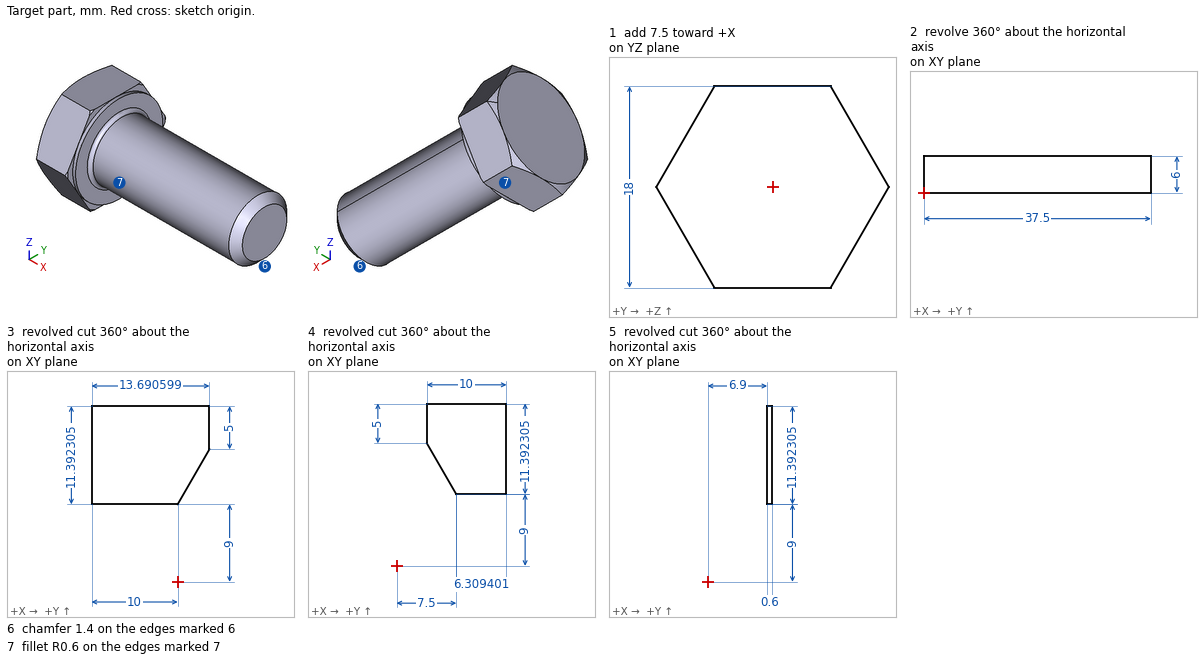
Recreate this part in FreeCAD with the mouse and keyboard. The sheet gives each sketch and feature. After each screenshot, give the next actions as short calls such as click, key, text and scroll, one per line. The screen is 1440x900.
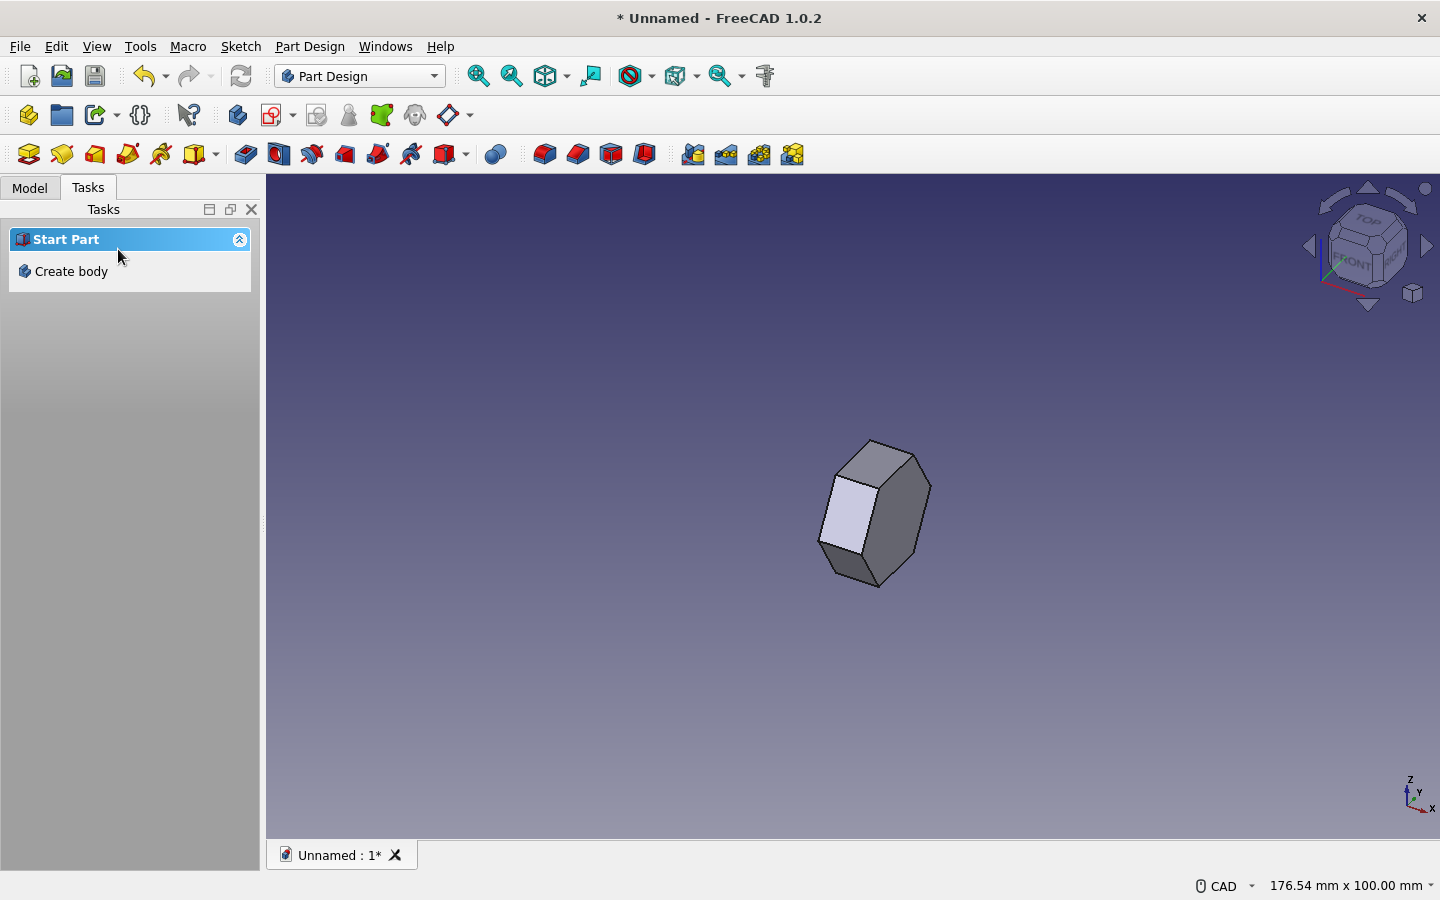
key(v)
key(f)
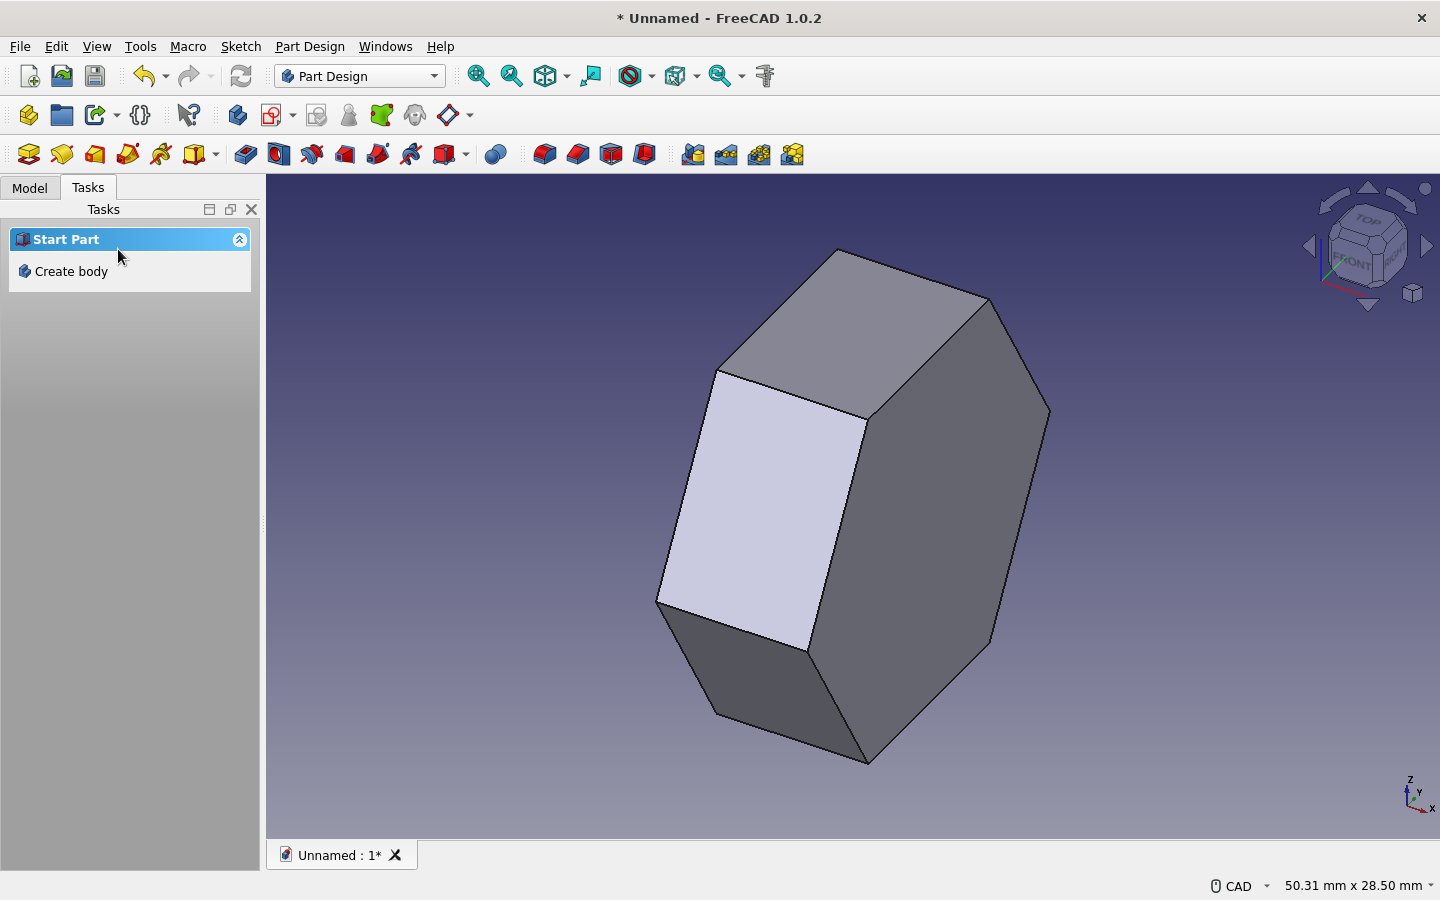
click(270, 116)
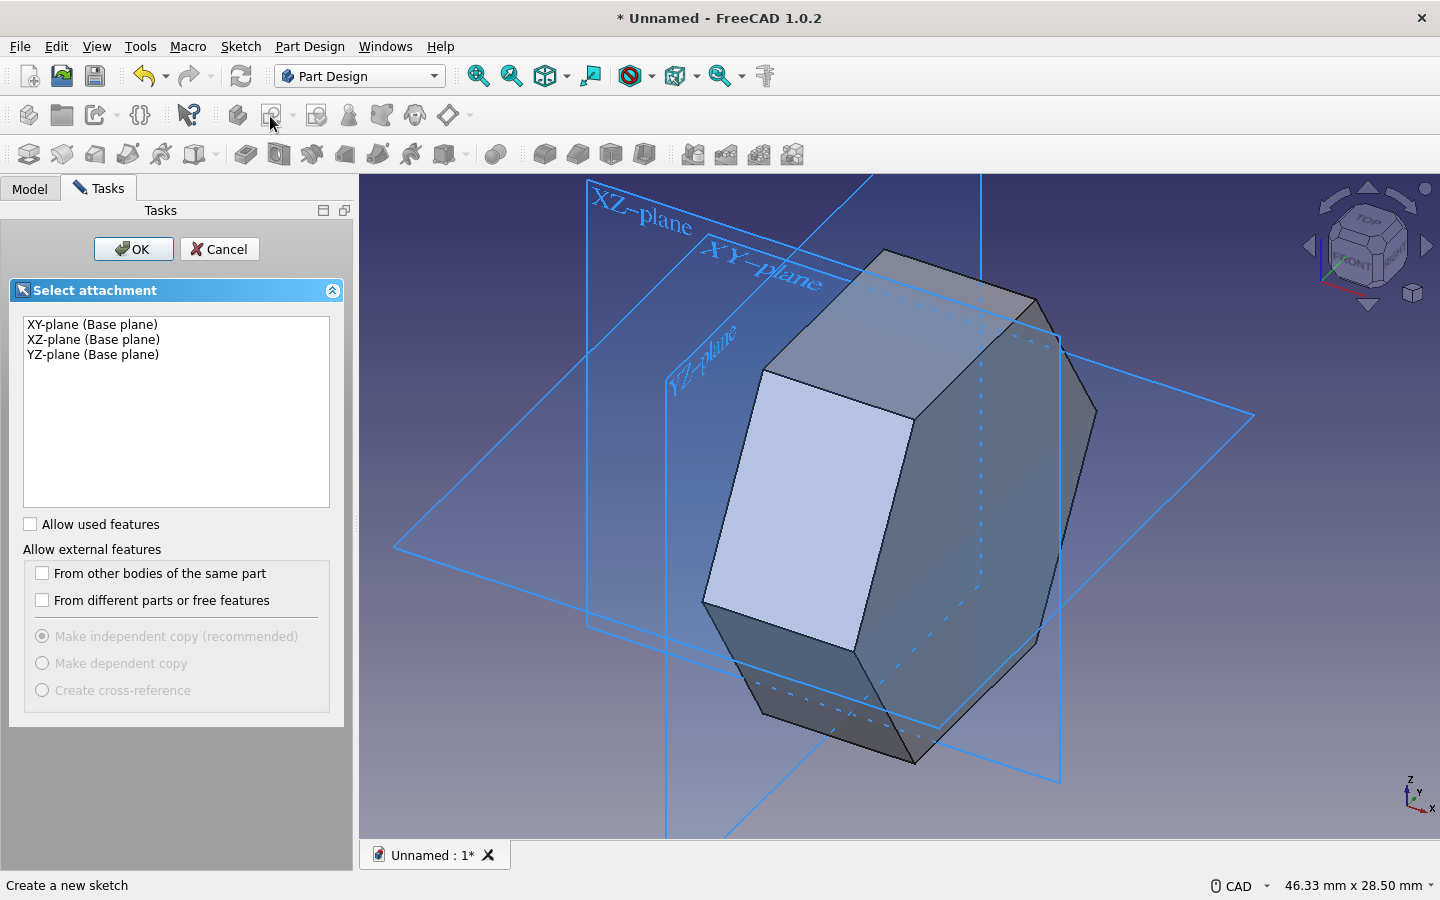
click(84, 324)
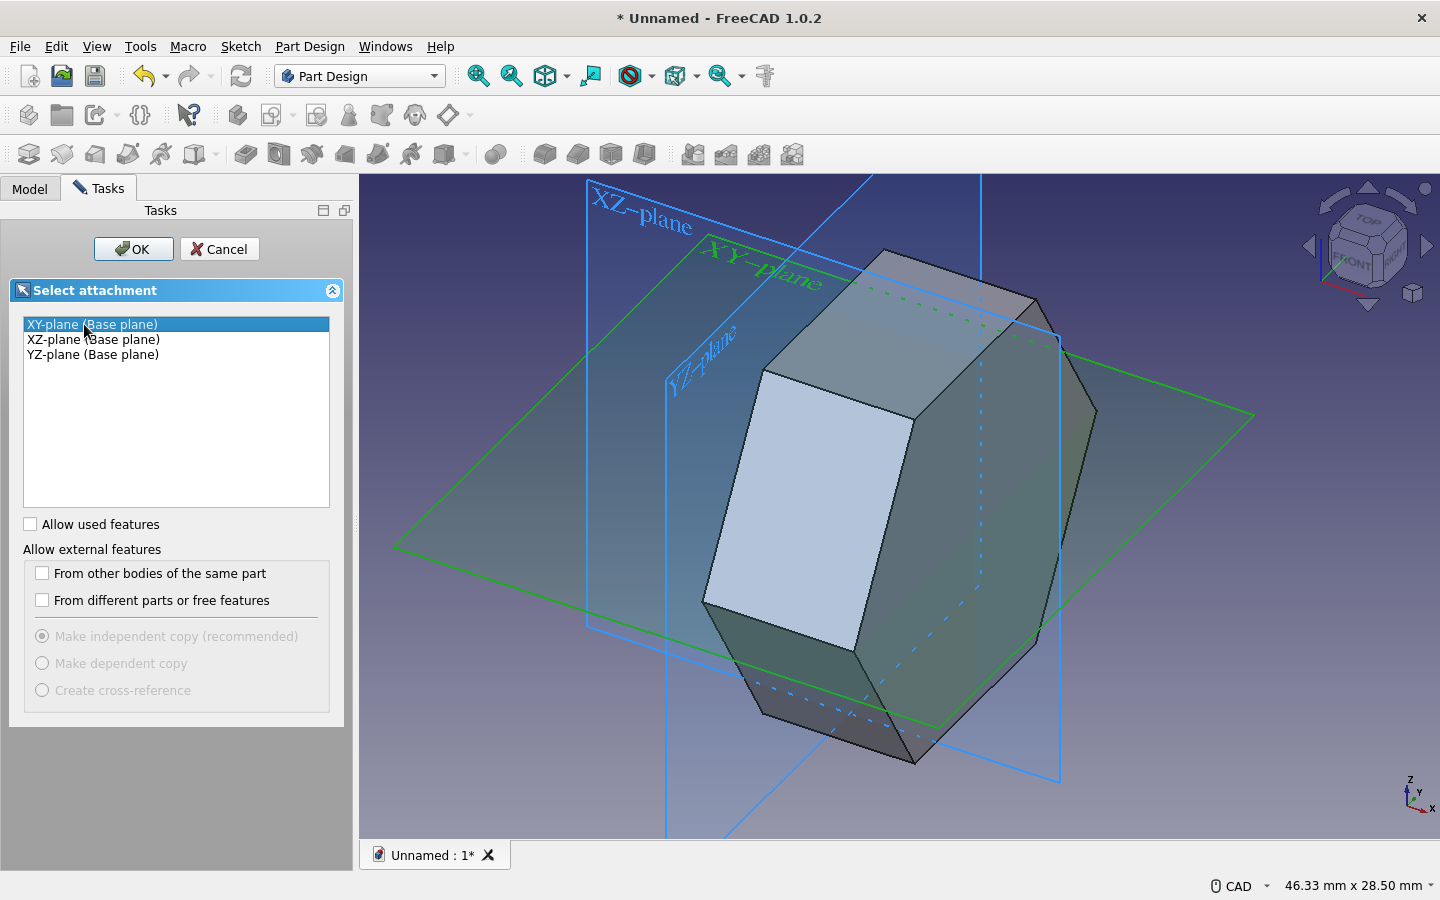
click(134, 249)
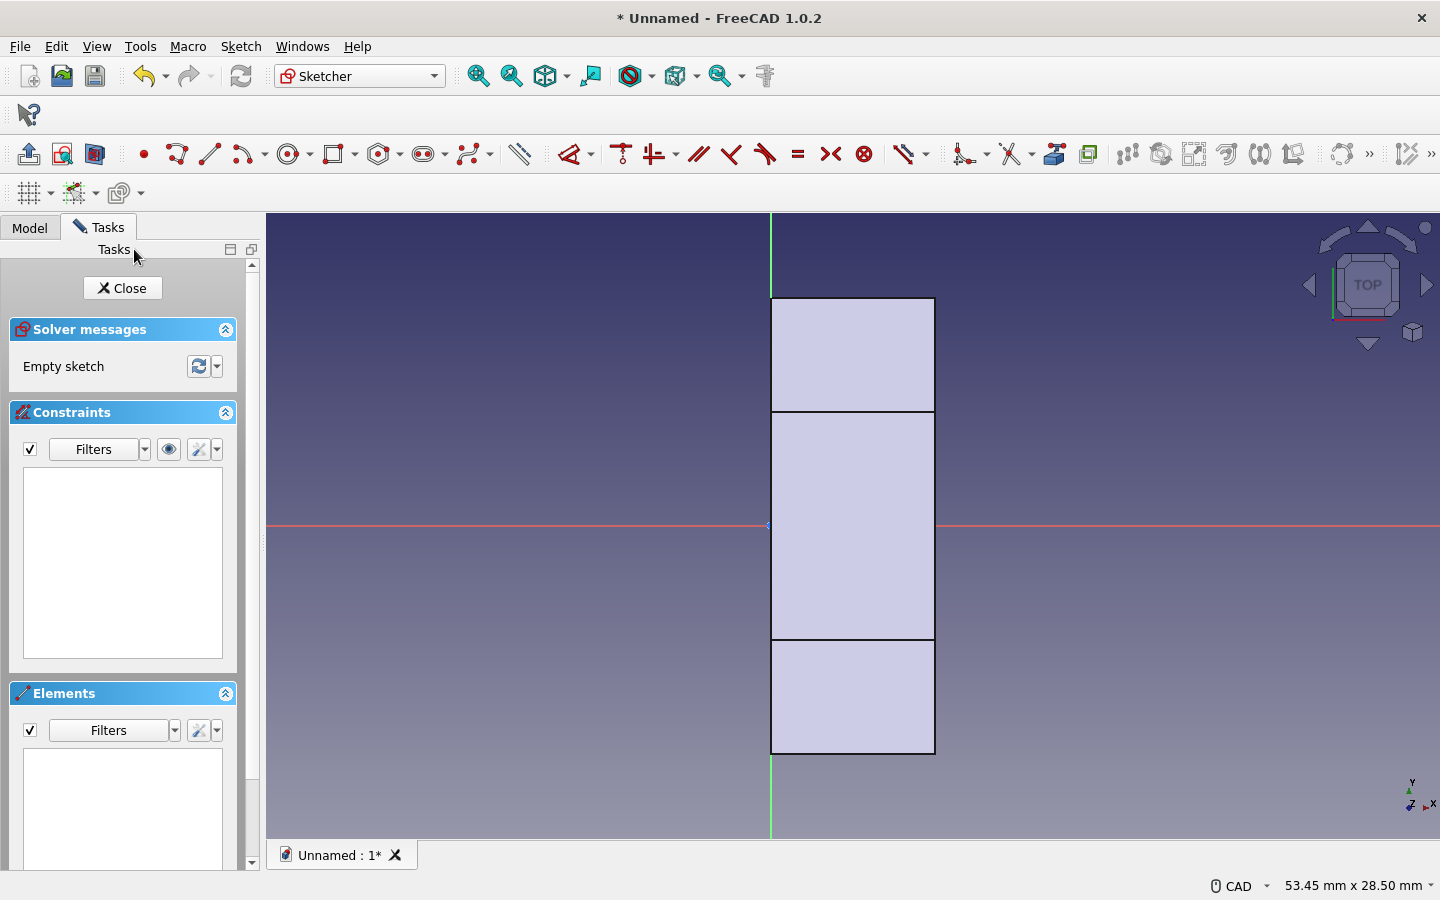
key(q)
key(s)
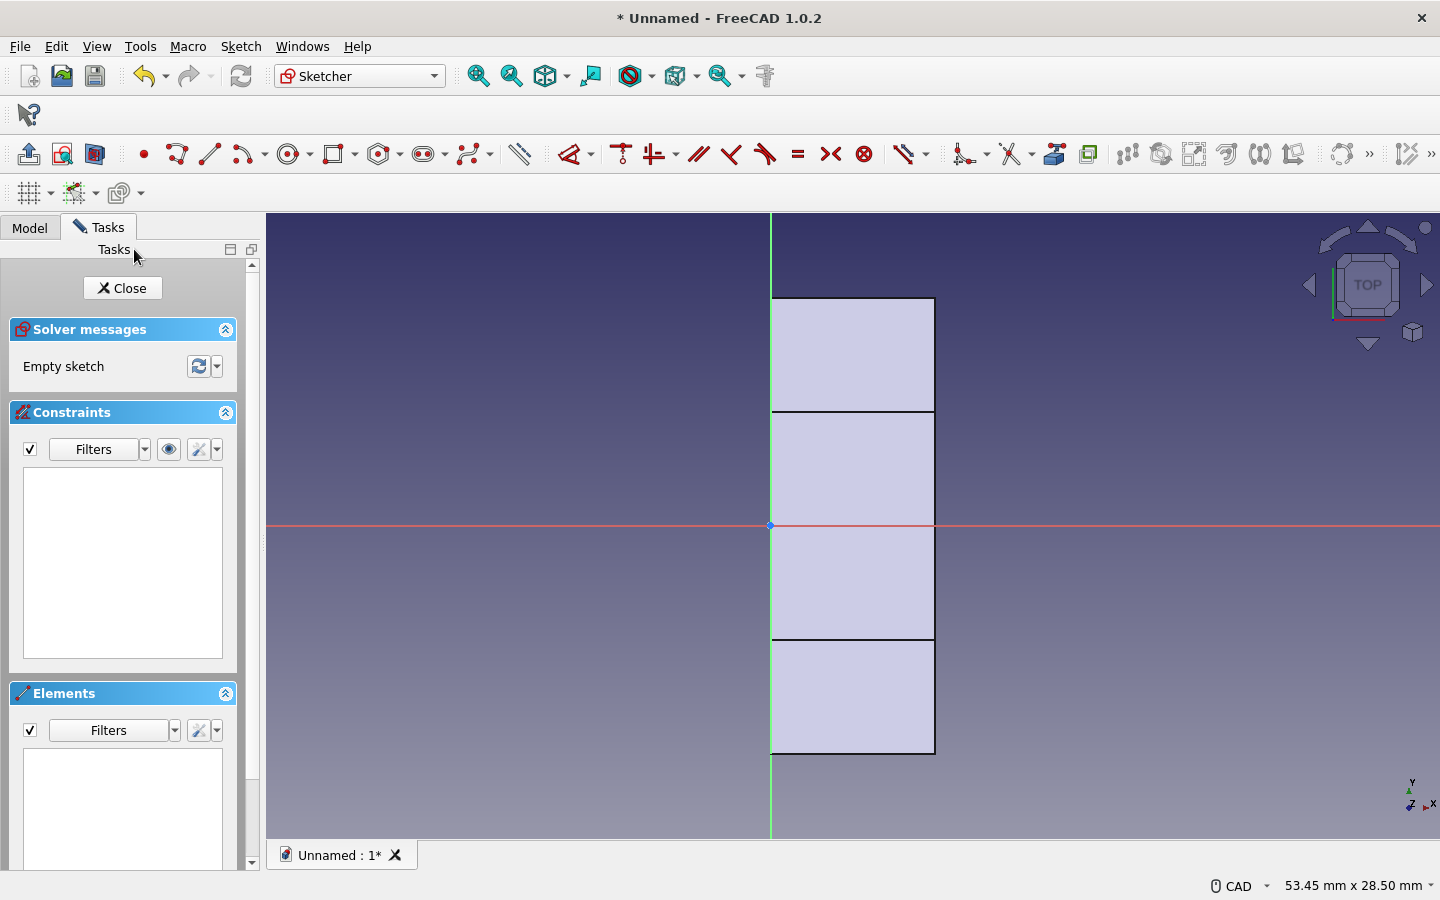
scroll(294, 660, down, 2)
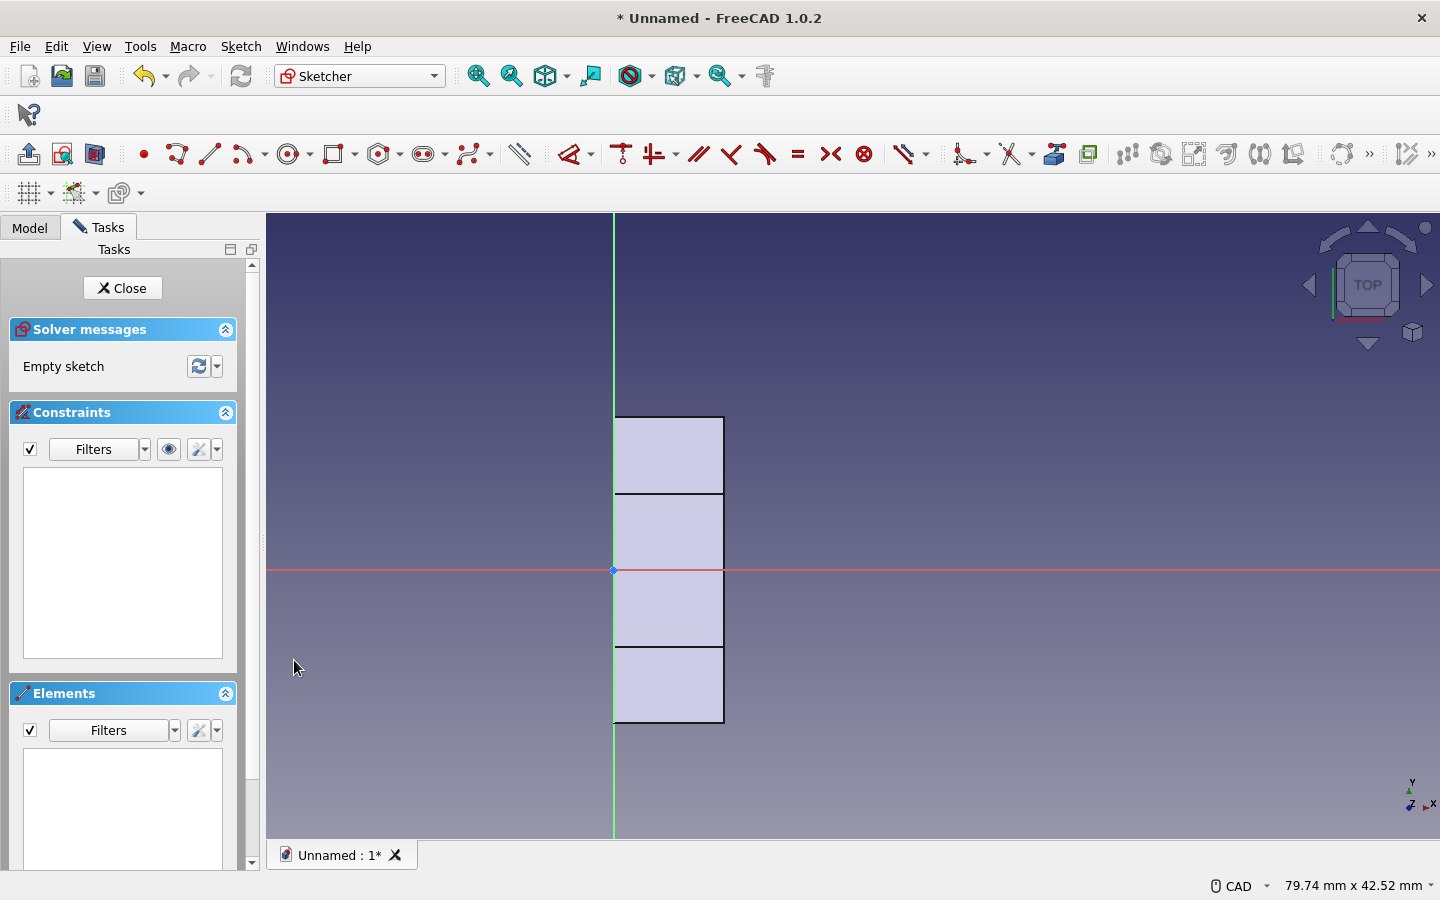
key(g)
key(r)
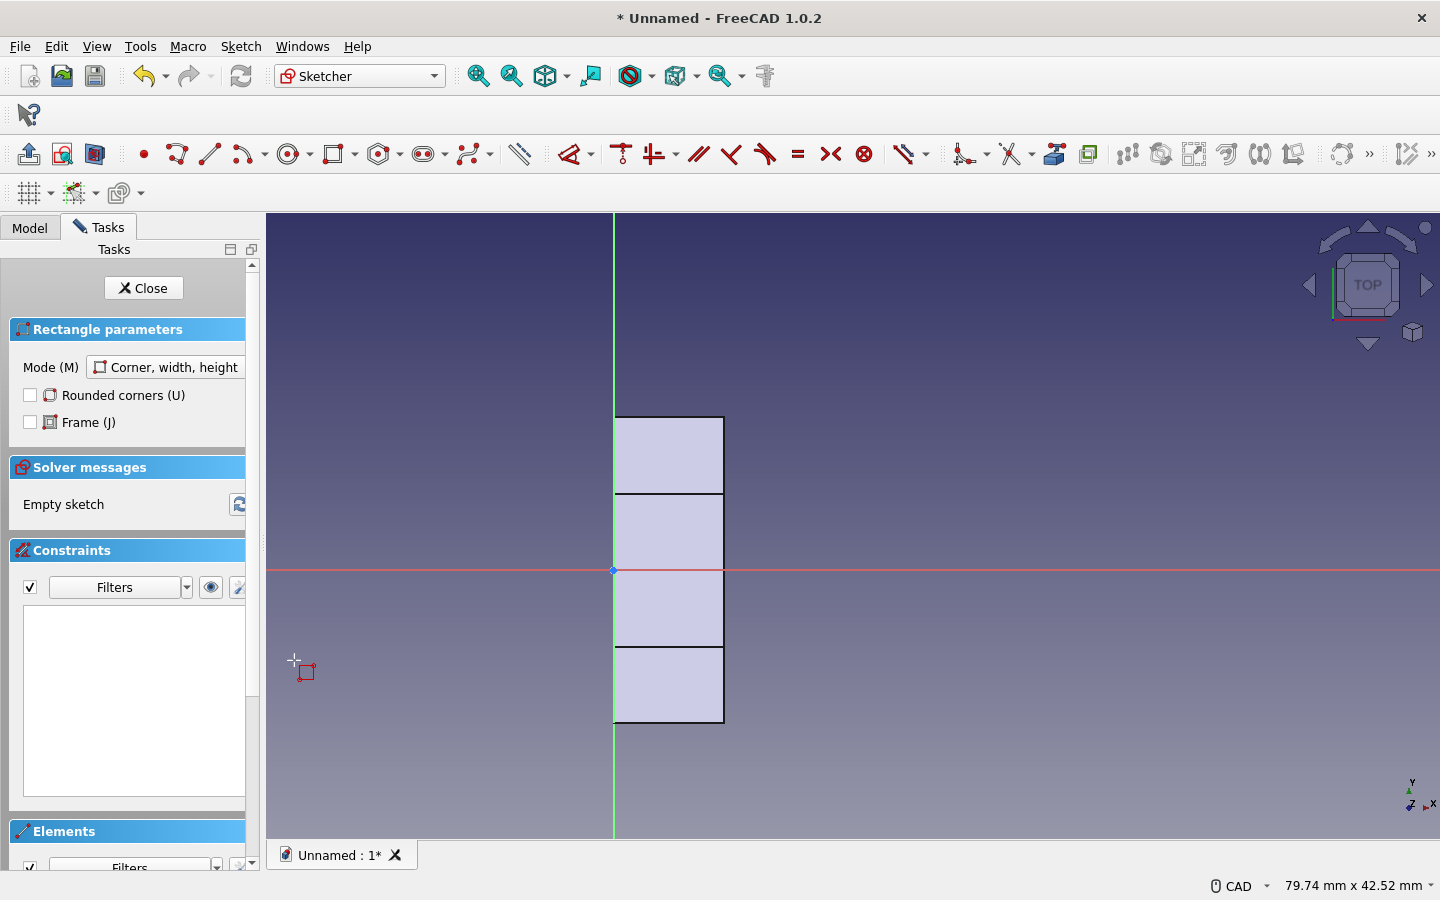
click(614, 570)
click(1166, 482)
key(Escape)